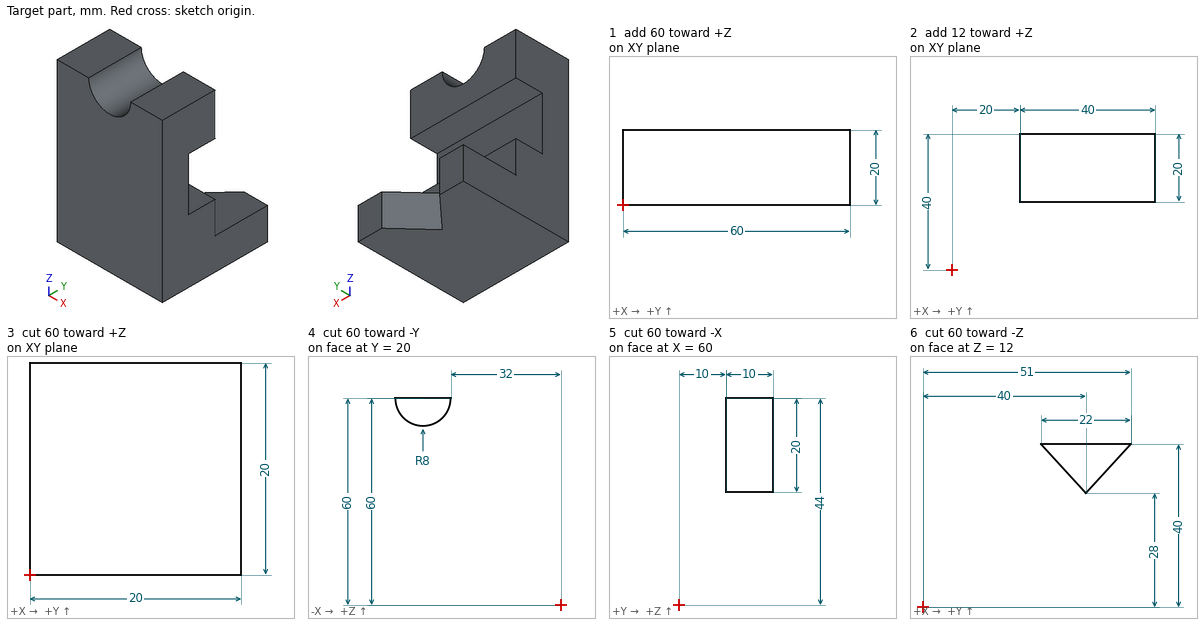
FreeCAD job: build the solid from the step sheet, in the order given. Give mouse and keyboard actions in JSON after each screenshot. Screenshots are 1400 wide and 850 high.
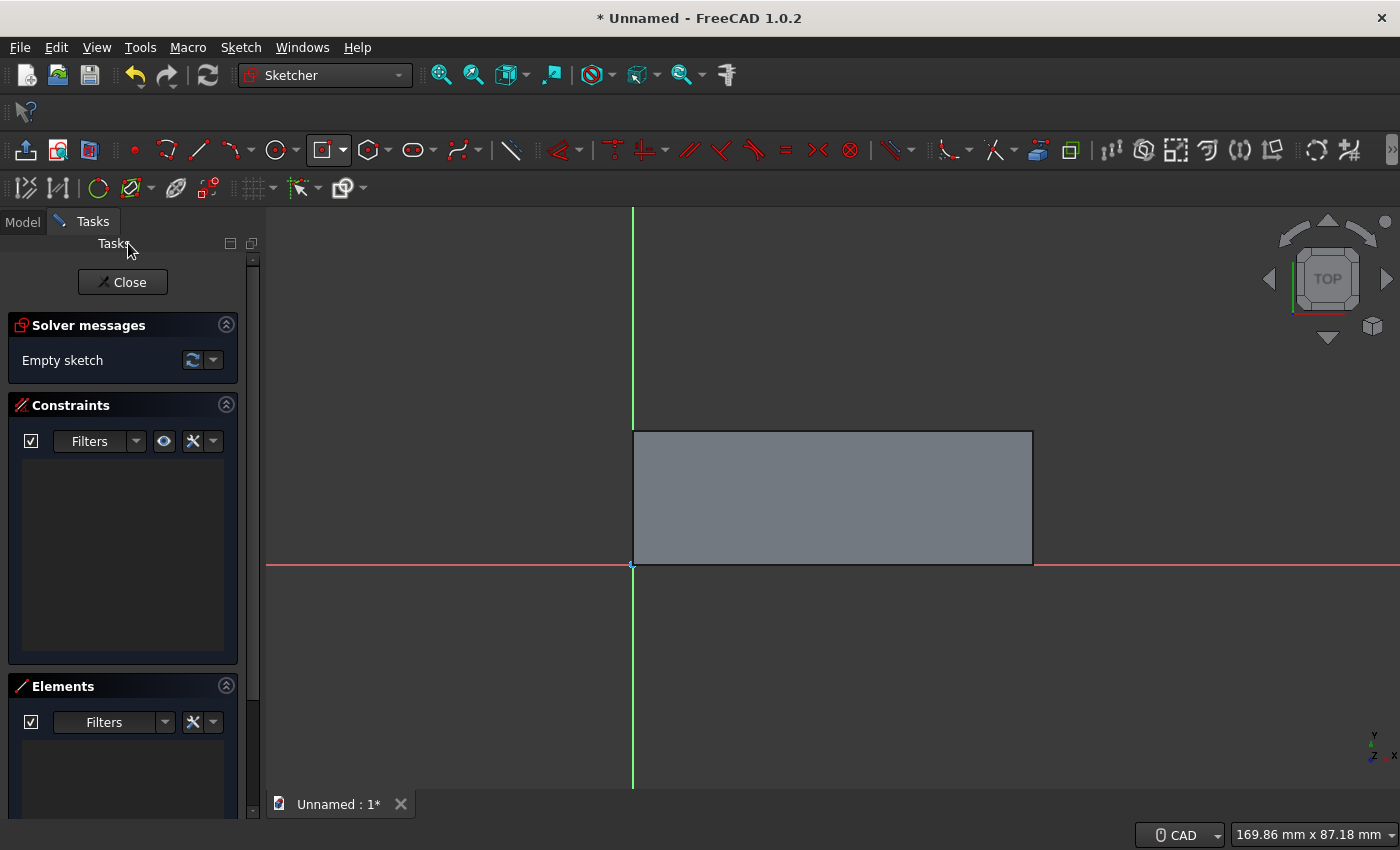
{"action": "left_click", "coordinate": [90, 150]}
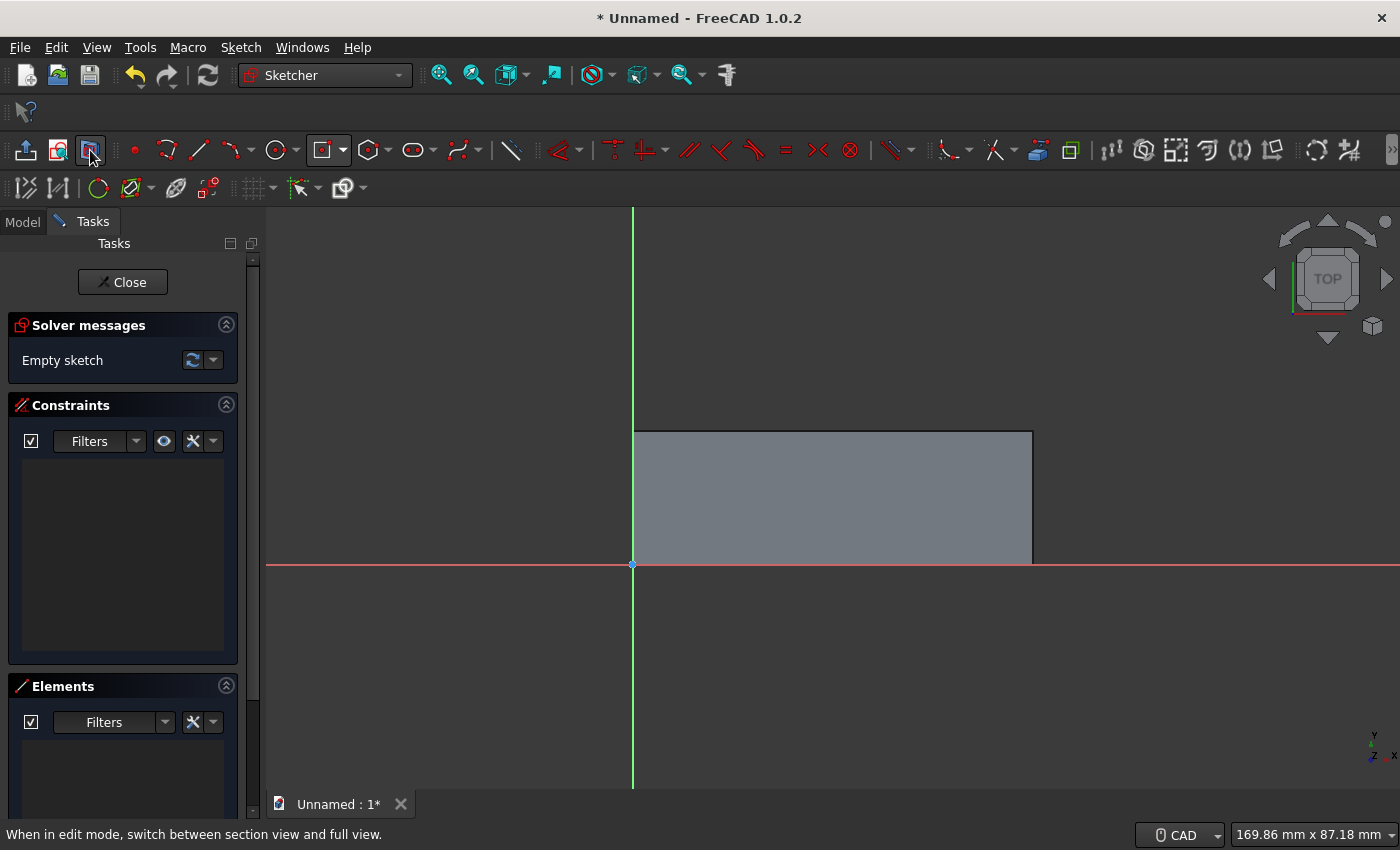
{"action": "scroll", "coordinate": [972, 296], "scroll_direction": "up", "scroll_amount": 2}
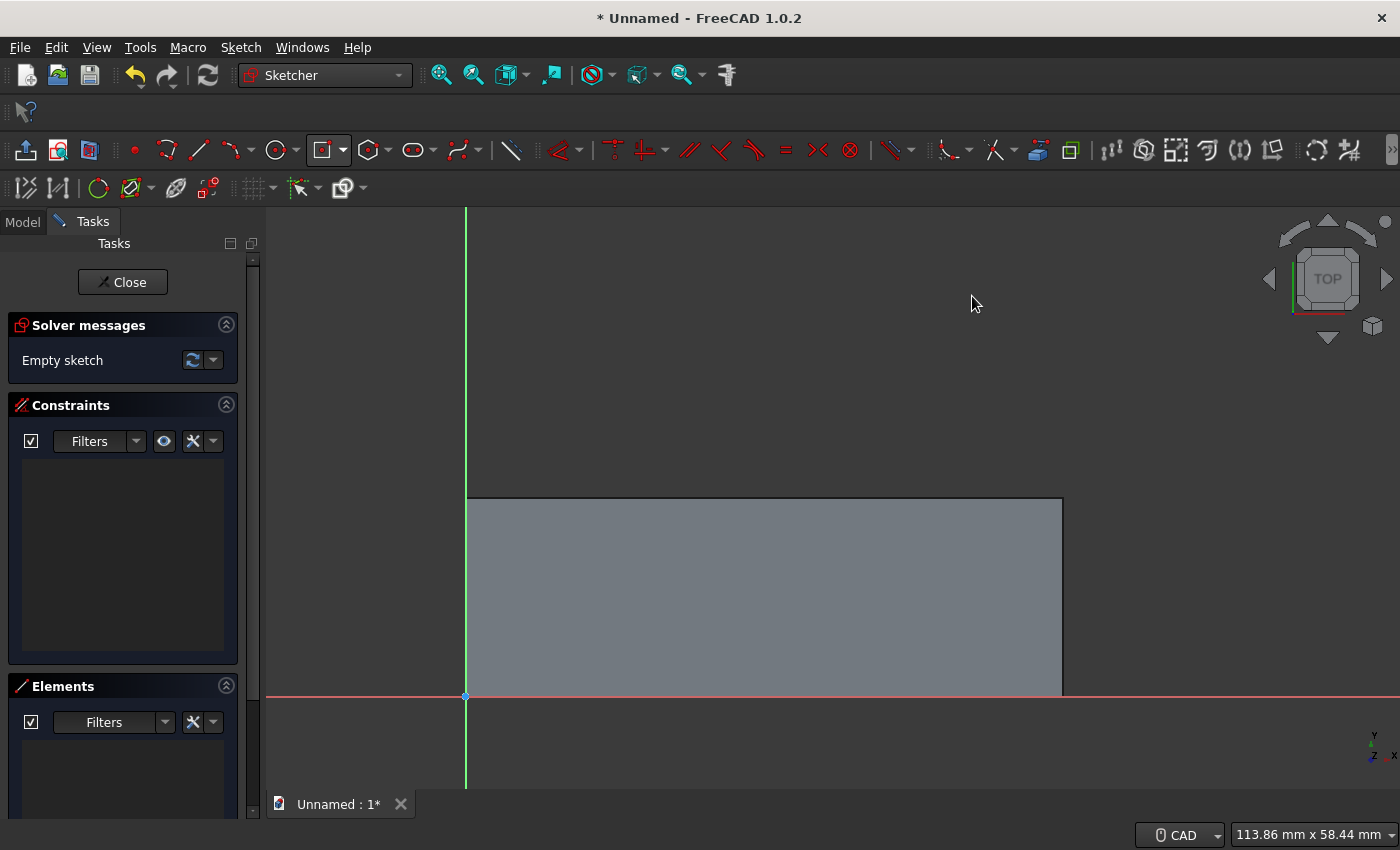
{"action": "left_click", "coordinate": [346, 150]}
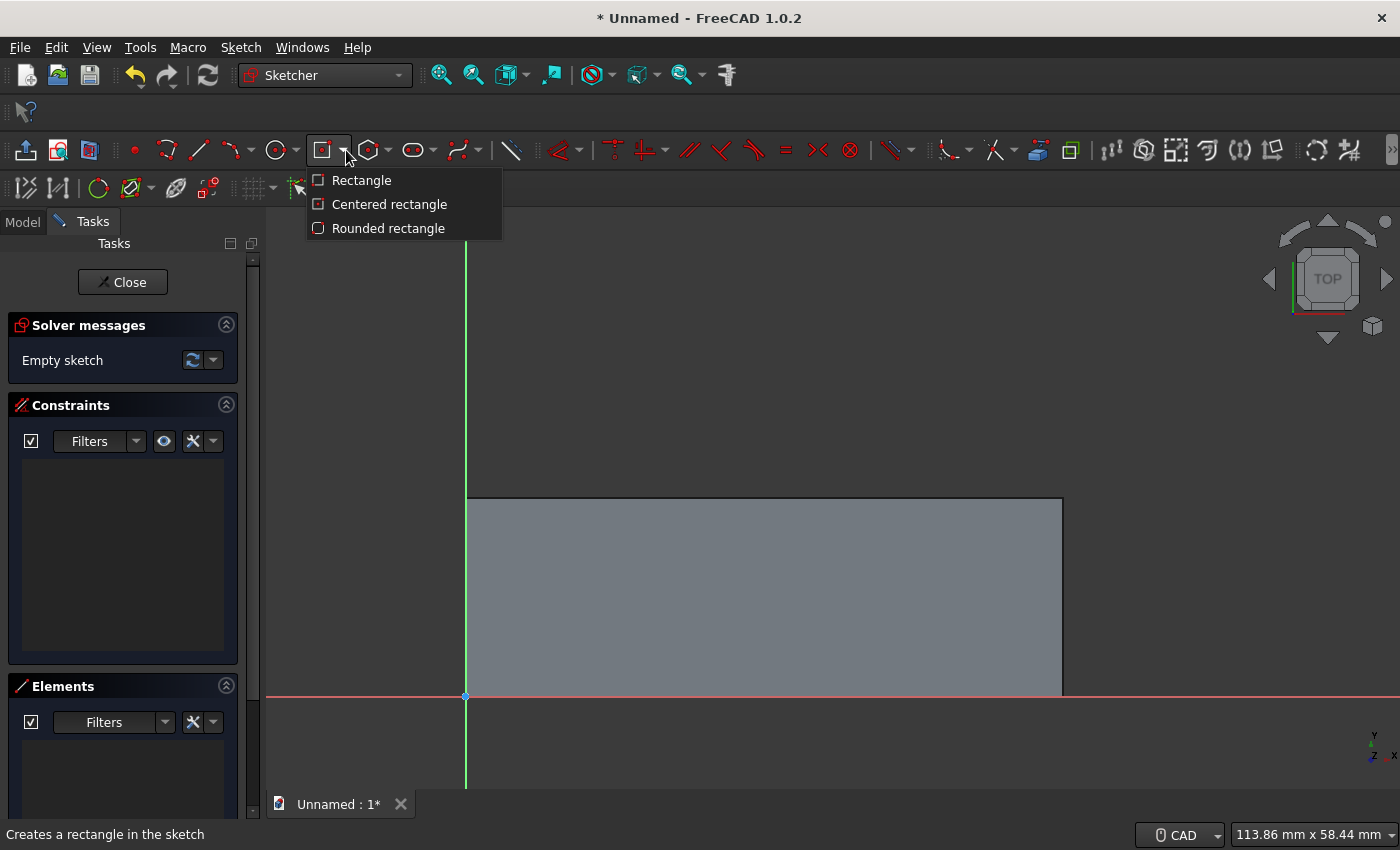
{"action": "left_click", "coordinate": [404, 180]}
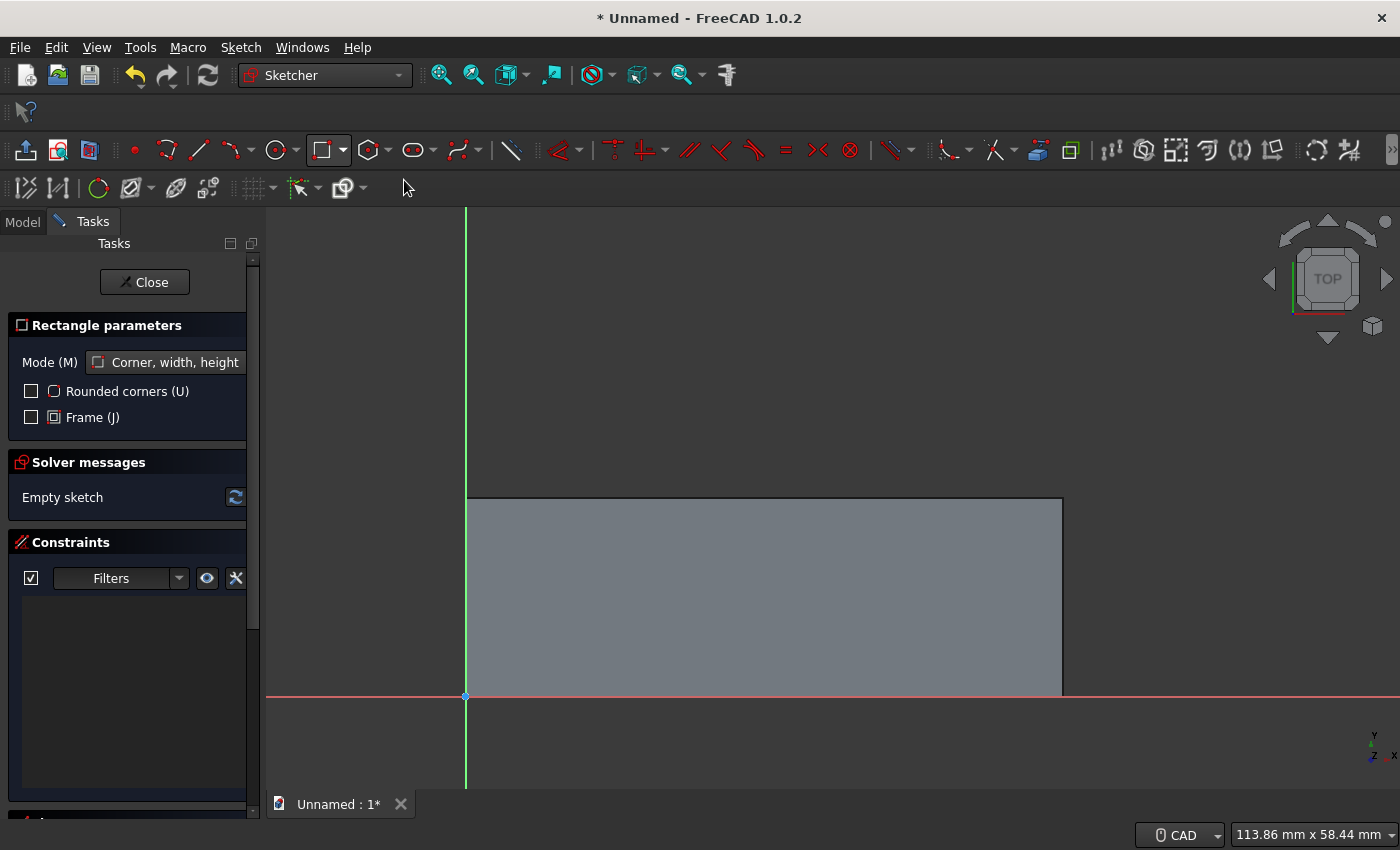
{"action": "left_click", "coordinate": [665, 298]}
{"action": "mouse_move", "coordinate": [1063, 498]}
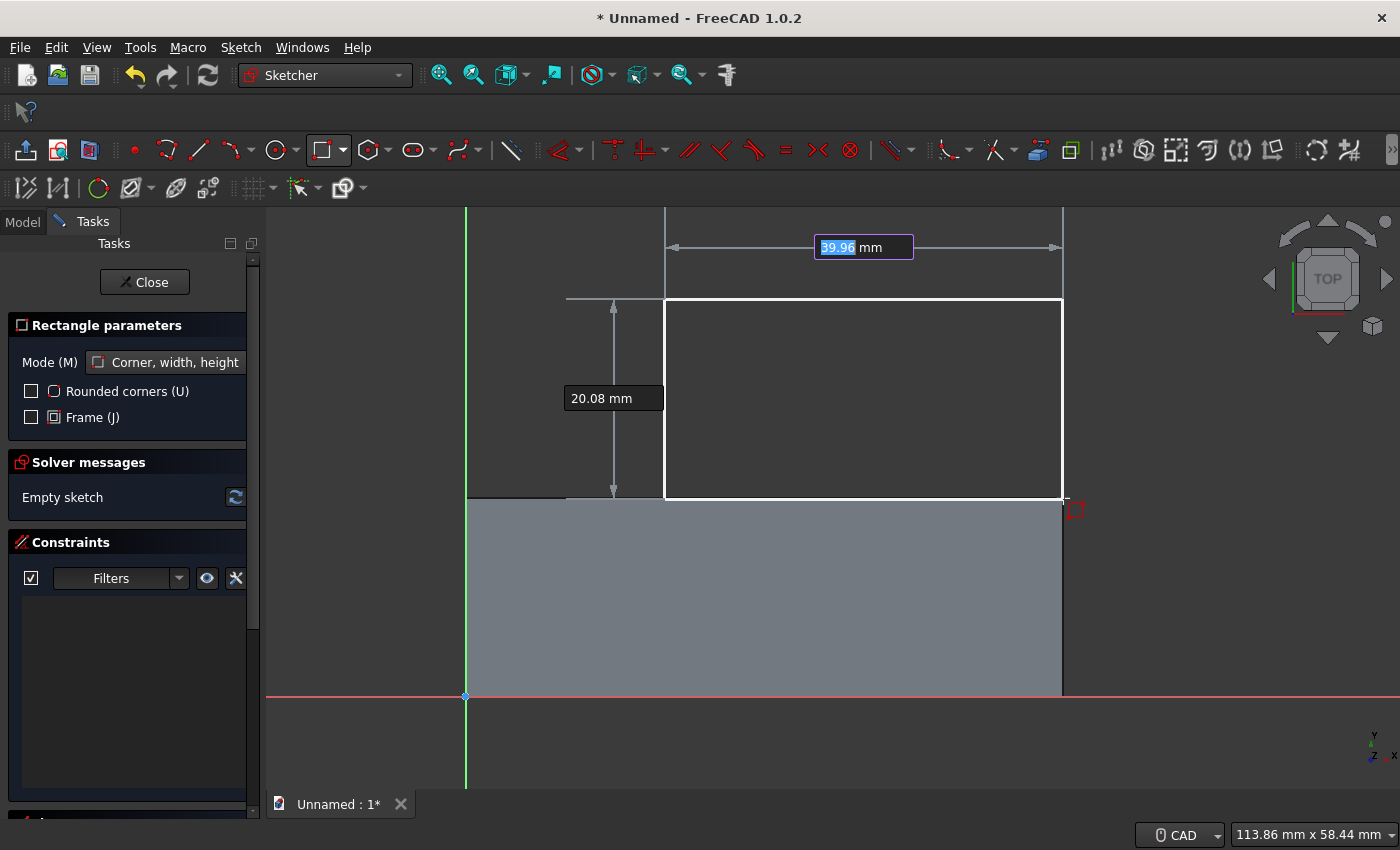
{"action": "type", "text": "40"}
{"action": "key", "text": "Tab"}
{"action": "type", "text": "20"}
{"action": "key", "text": "Return"}
{"action": "key", "text": "Escape"}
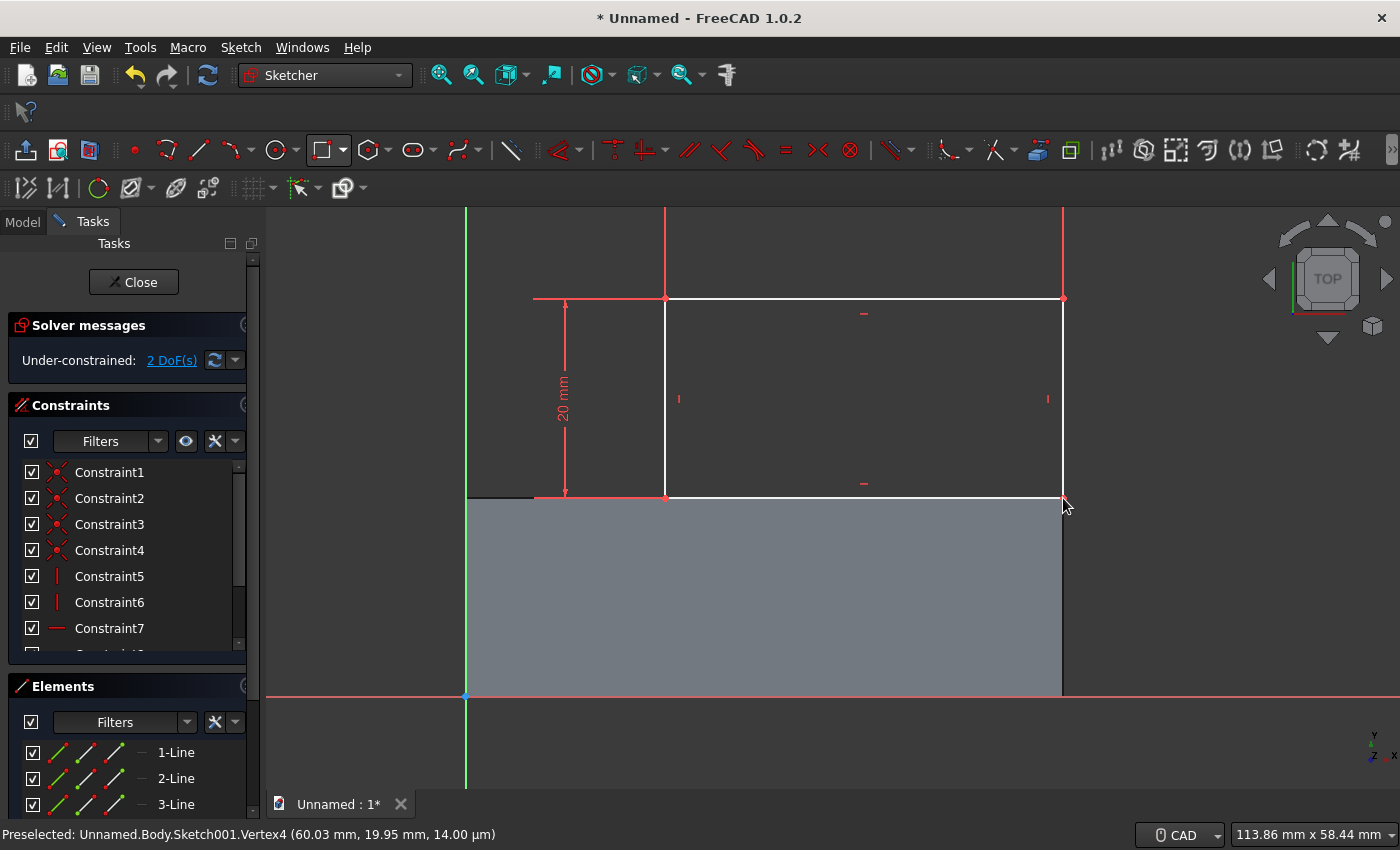
{"action": "left_click", "coordinate": [558, 150]}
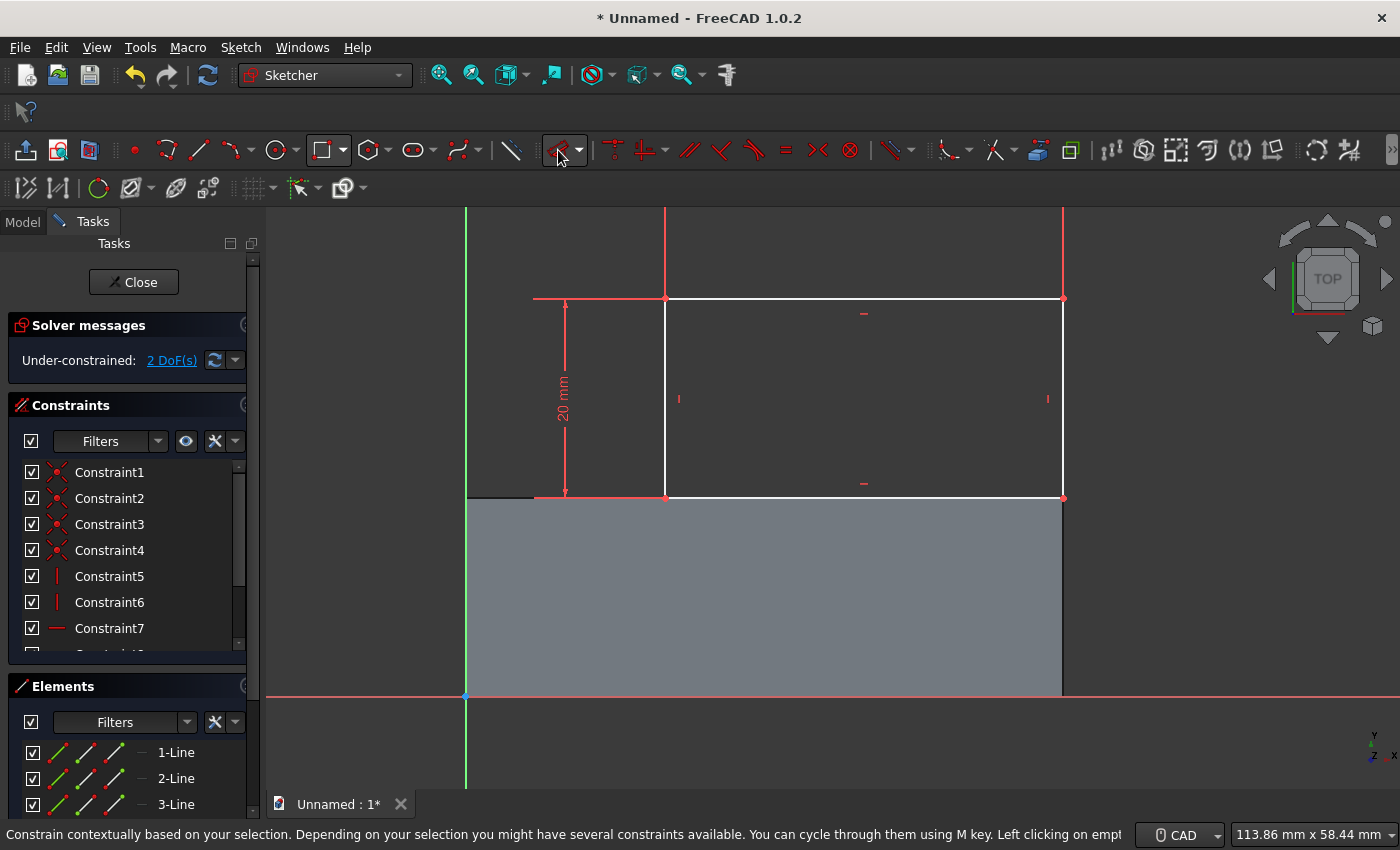
{"action": "left_click", "coordinate": [665, 299]}
{"action": "left_click", "coordinate": [565, 731]}